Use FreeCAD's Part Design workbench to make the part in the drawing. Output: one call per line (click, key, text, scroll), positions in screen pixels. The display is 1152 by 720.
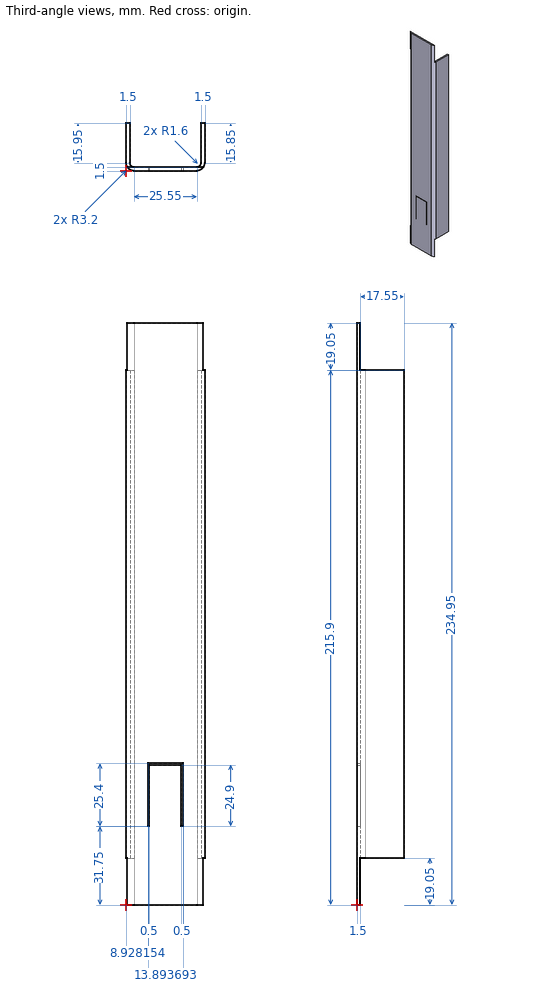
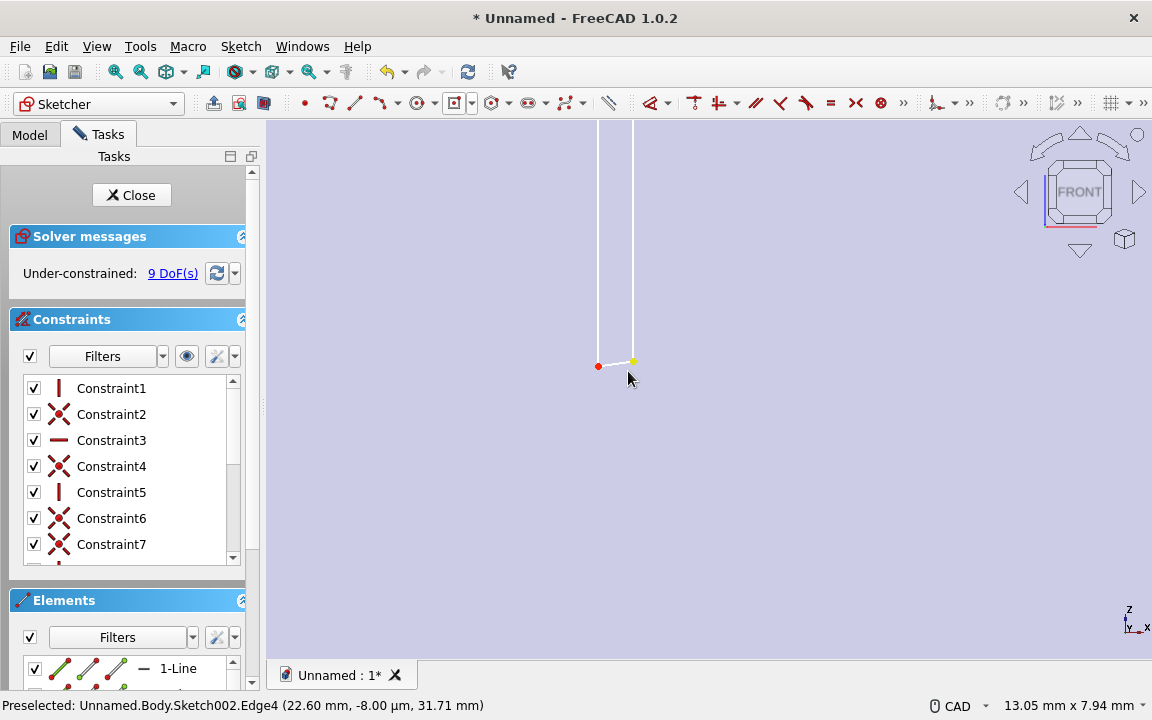
click(619, 363)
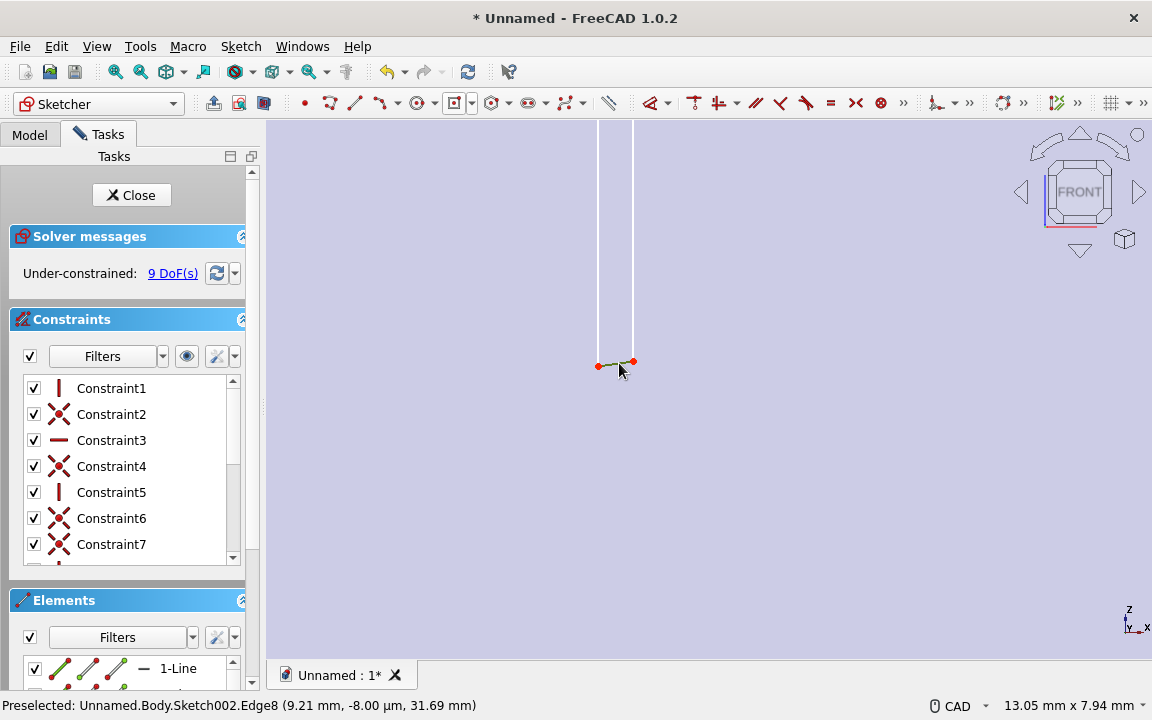
key(h)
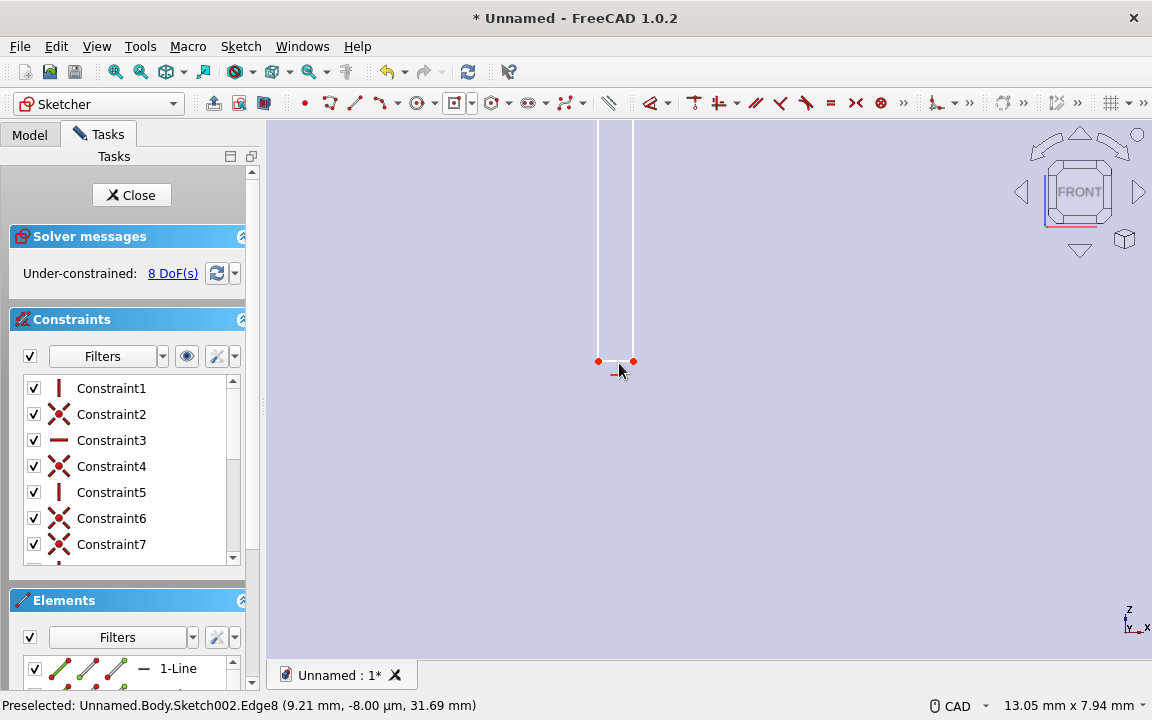
click(650, 104)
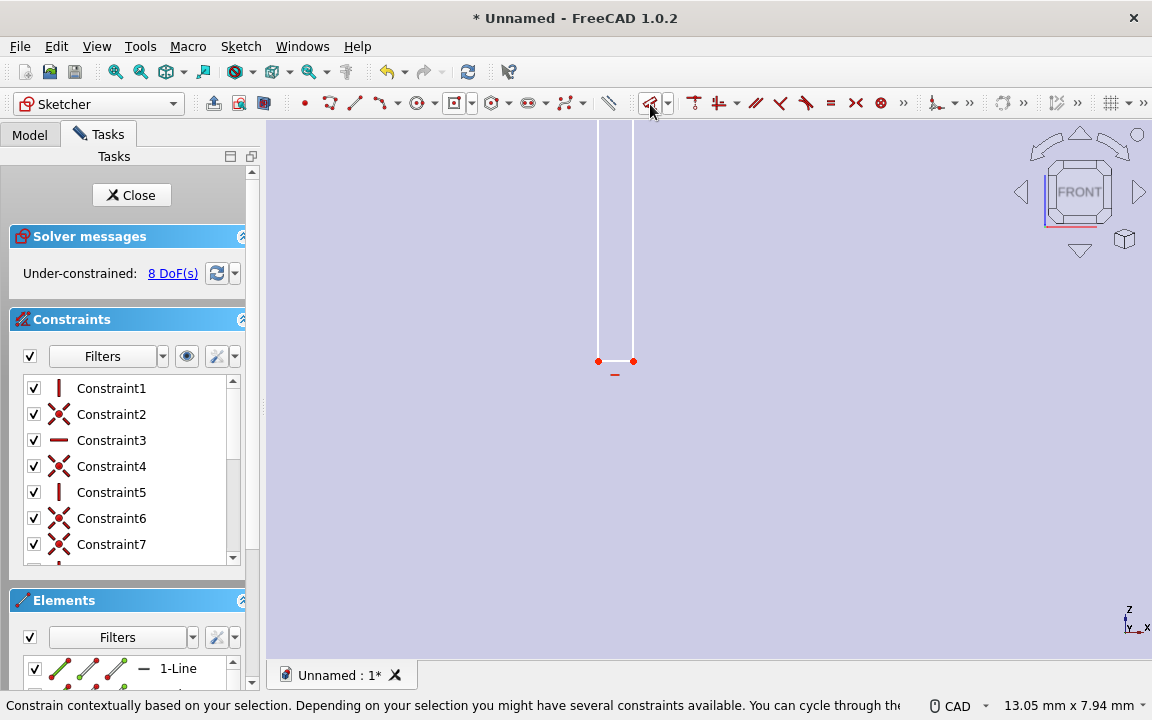
scroll(628, 371, down, 12)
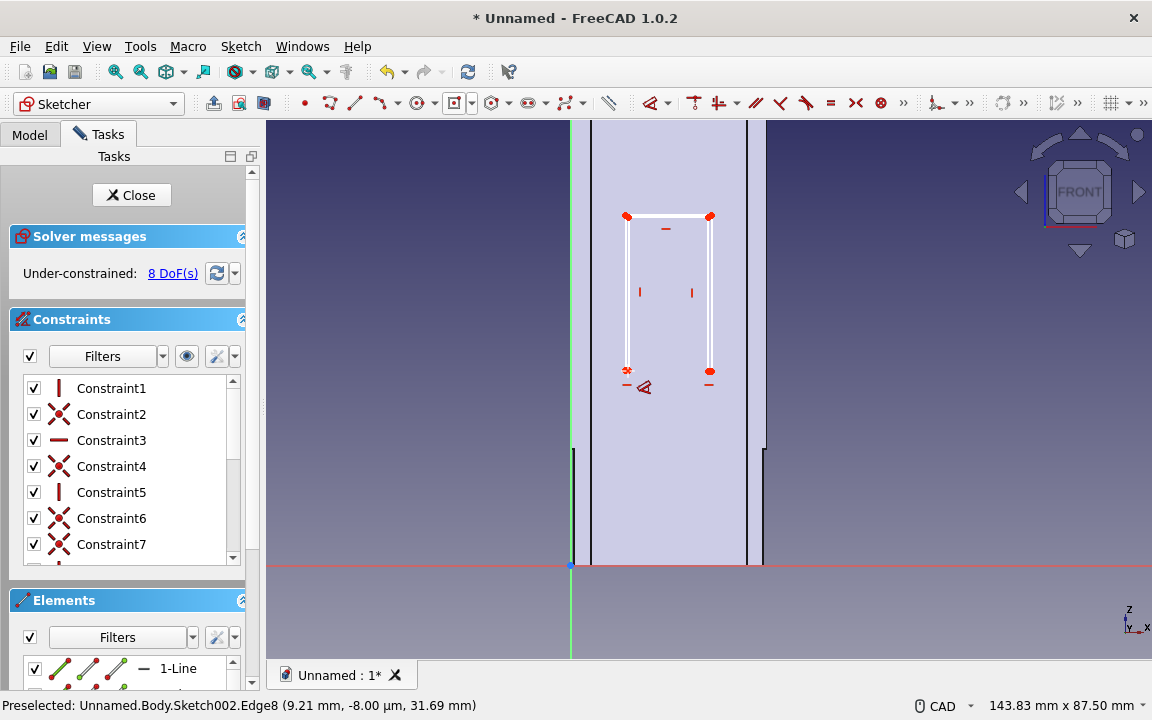
scroll(711, 371, up, 14)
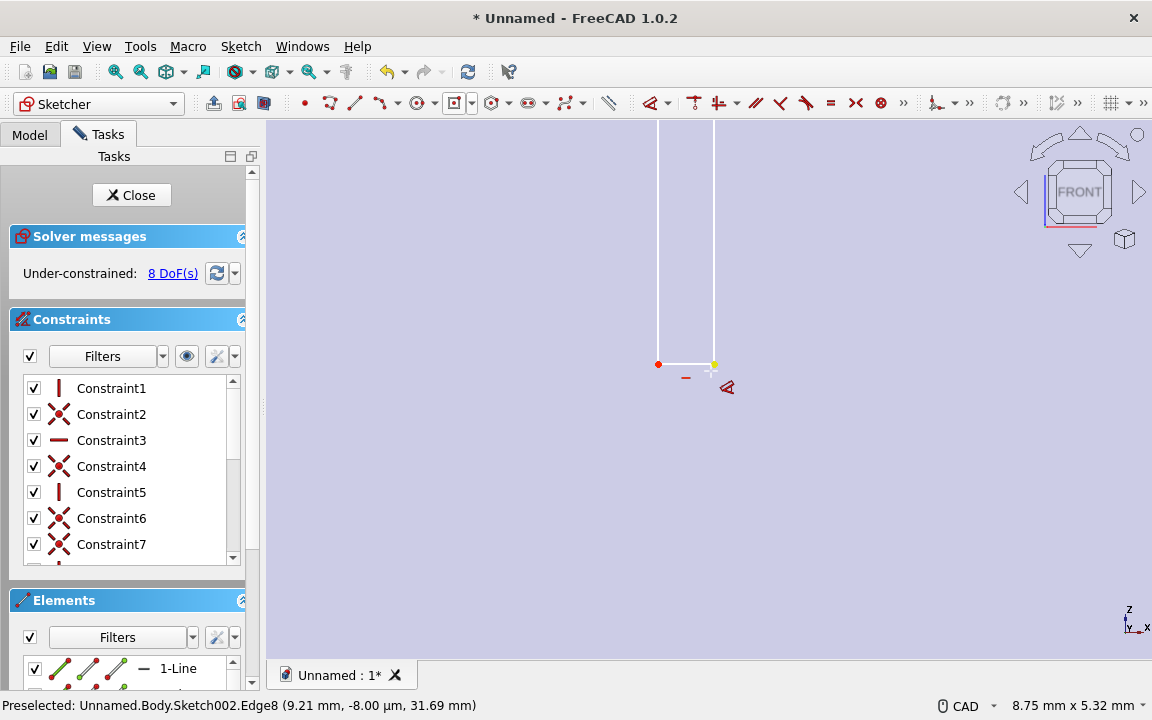
click(697, 364)
click(686, 330)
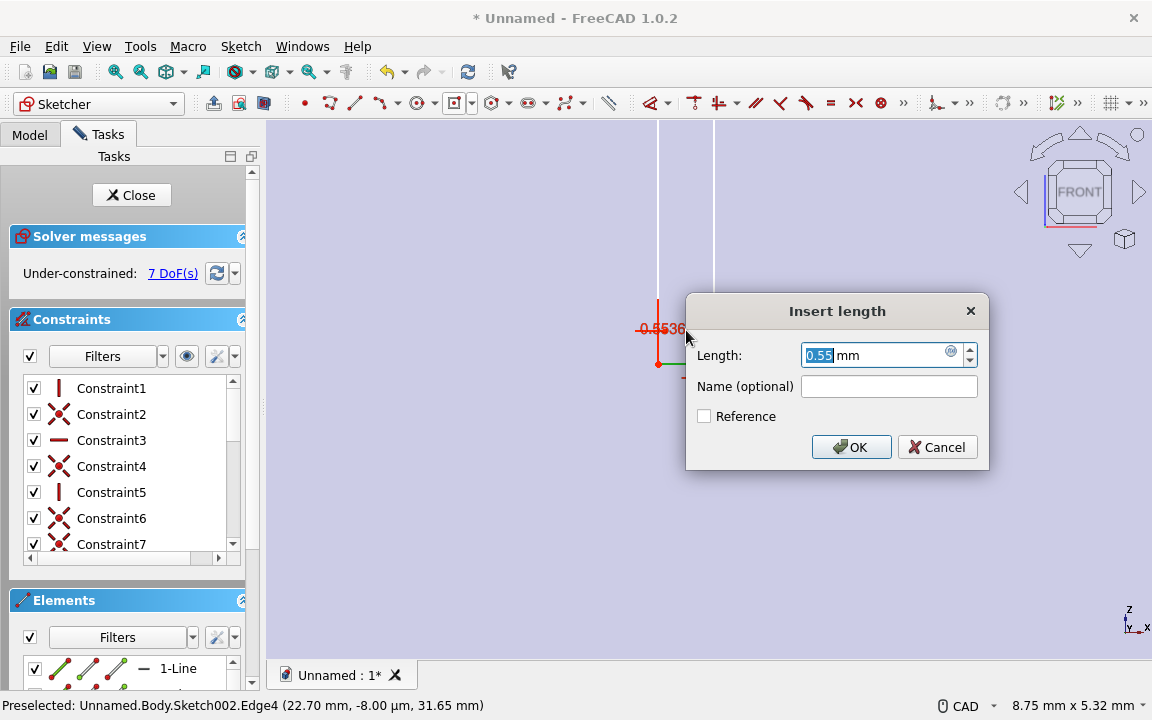
text(0.5)
key(Return)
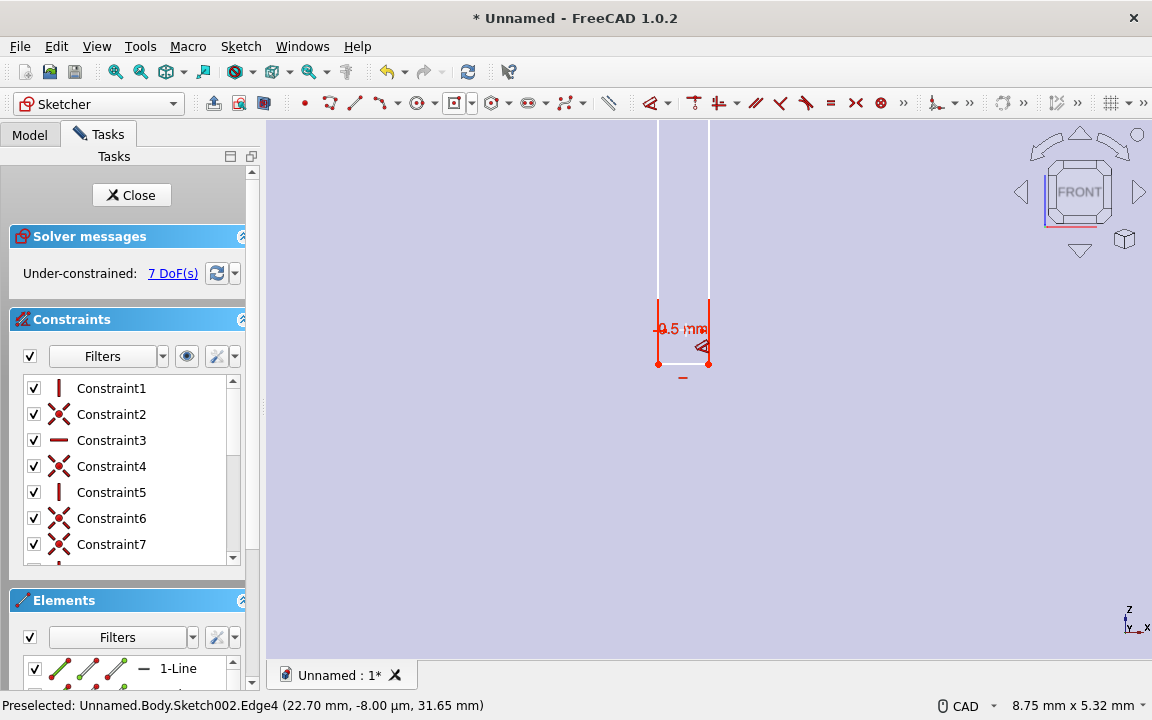
scroll(711, 371, down, 14)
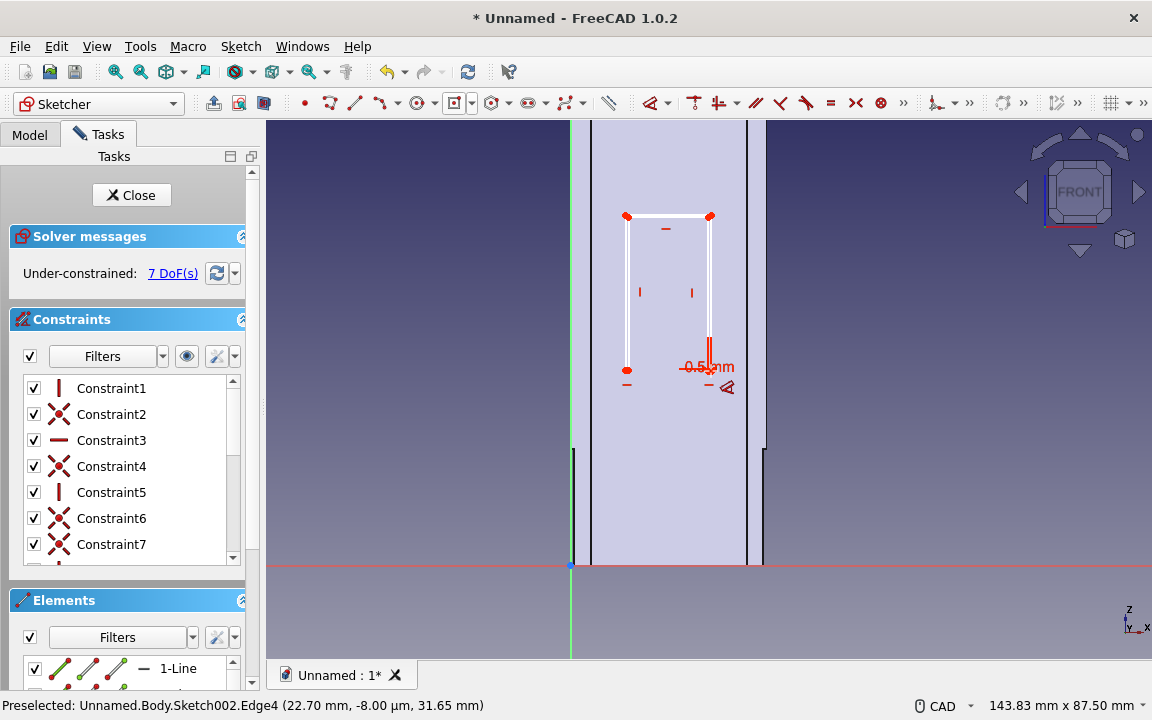
scroll(628, 371, up, 14)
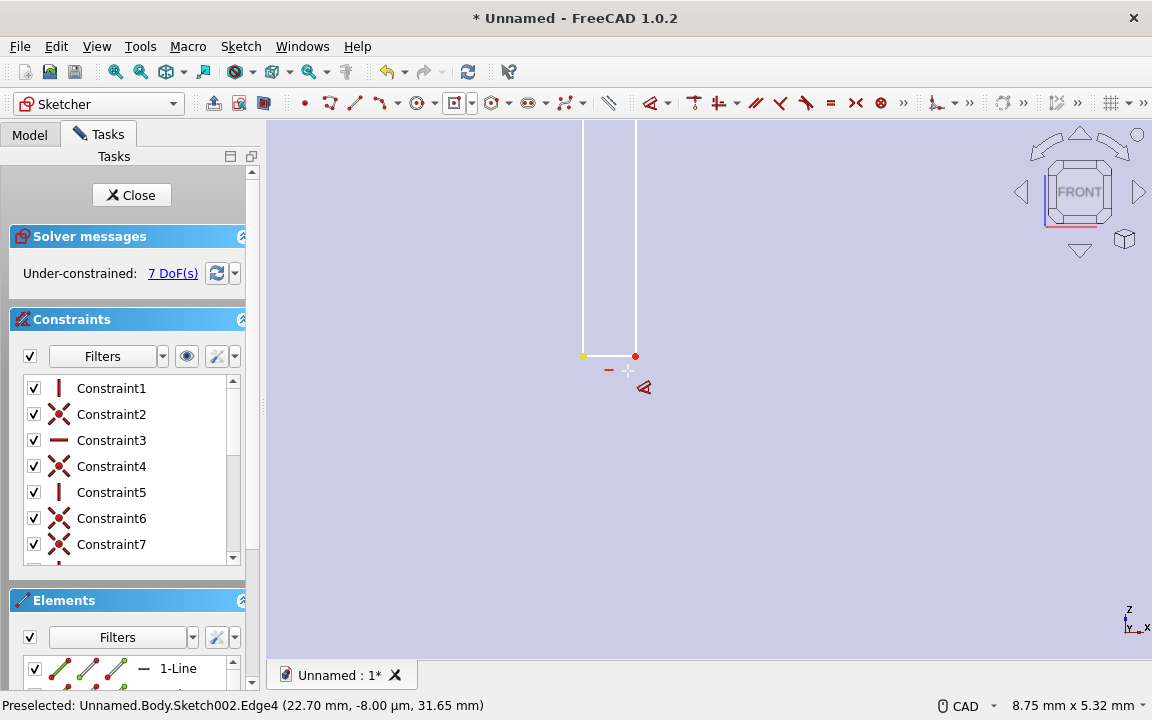
click(620, 356)
click(609, 322)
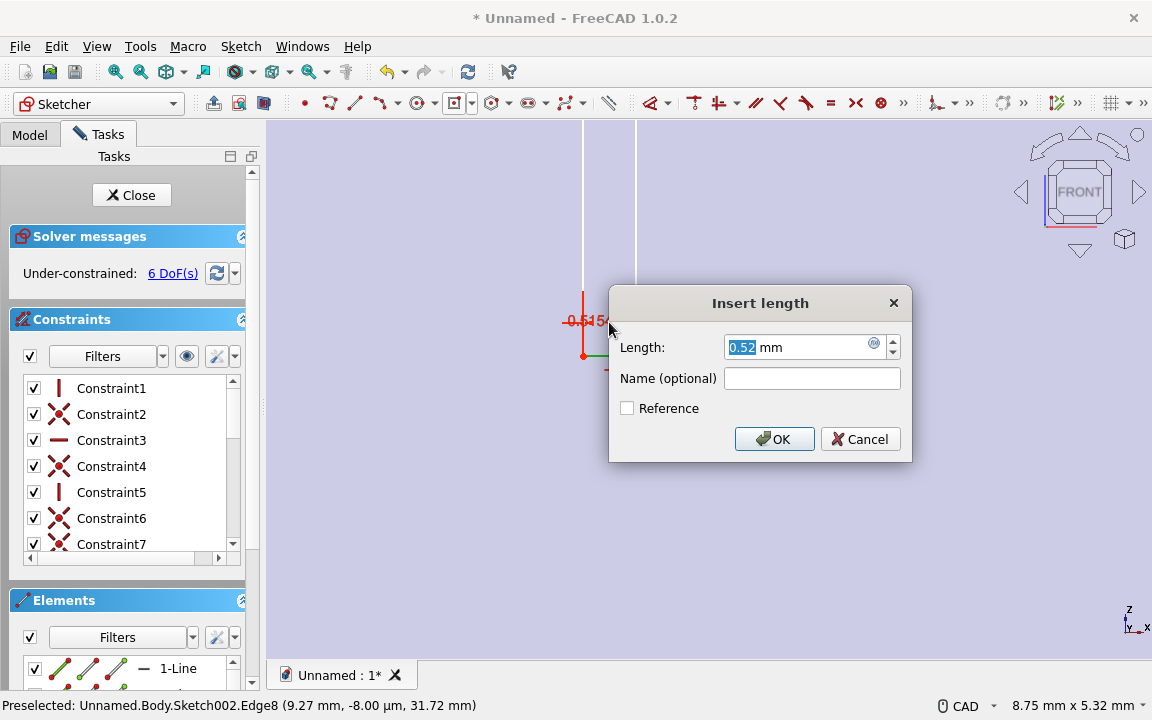
text(0.5)
key(Return)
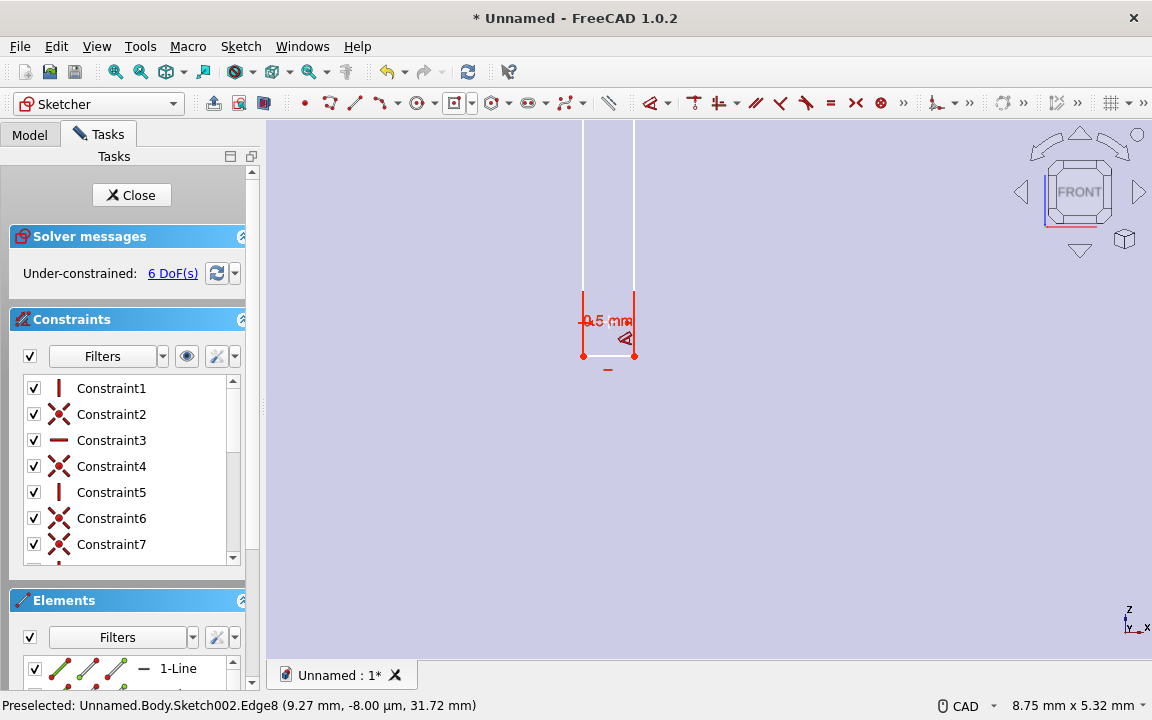
scroll(628, 371, down, 14)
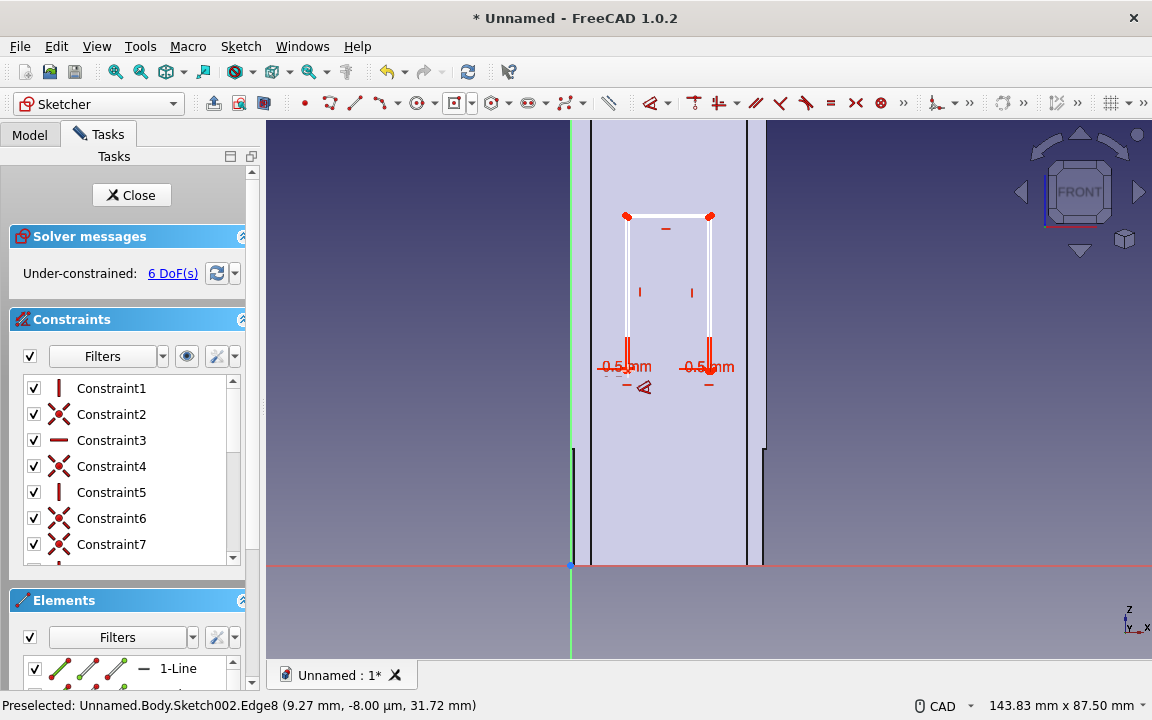
scroll(626, 324, up, 8)